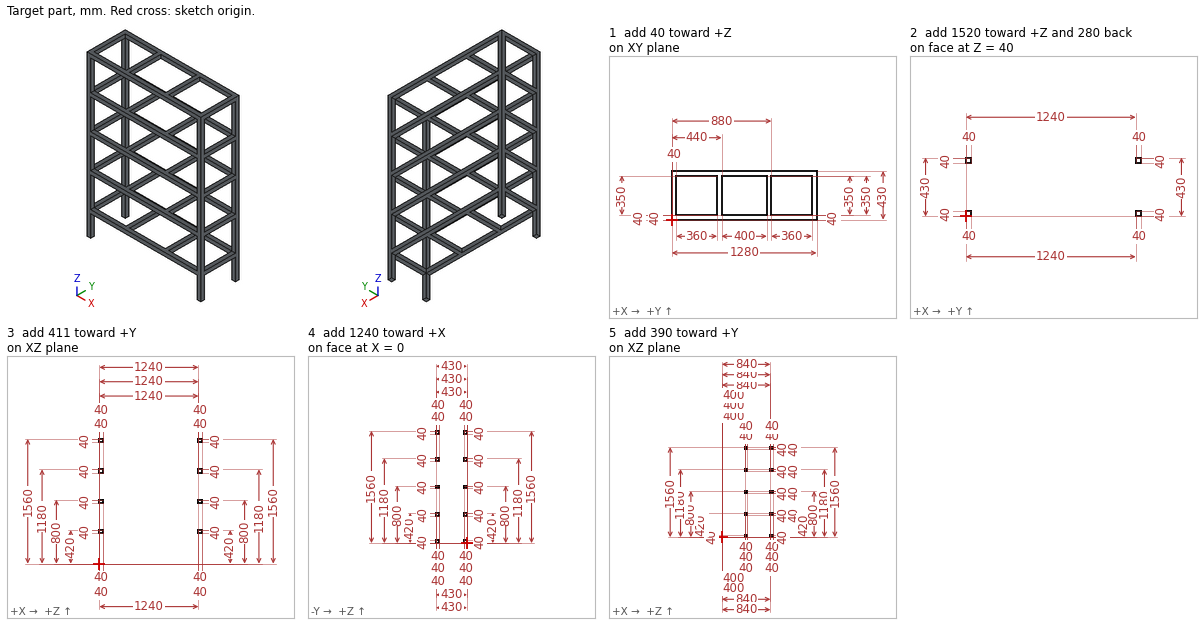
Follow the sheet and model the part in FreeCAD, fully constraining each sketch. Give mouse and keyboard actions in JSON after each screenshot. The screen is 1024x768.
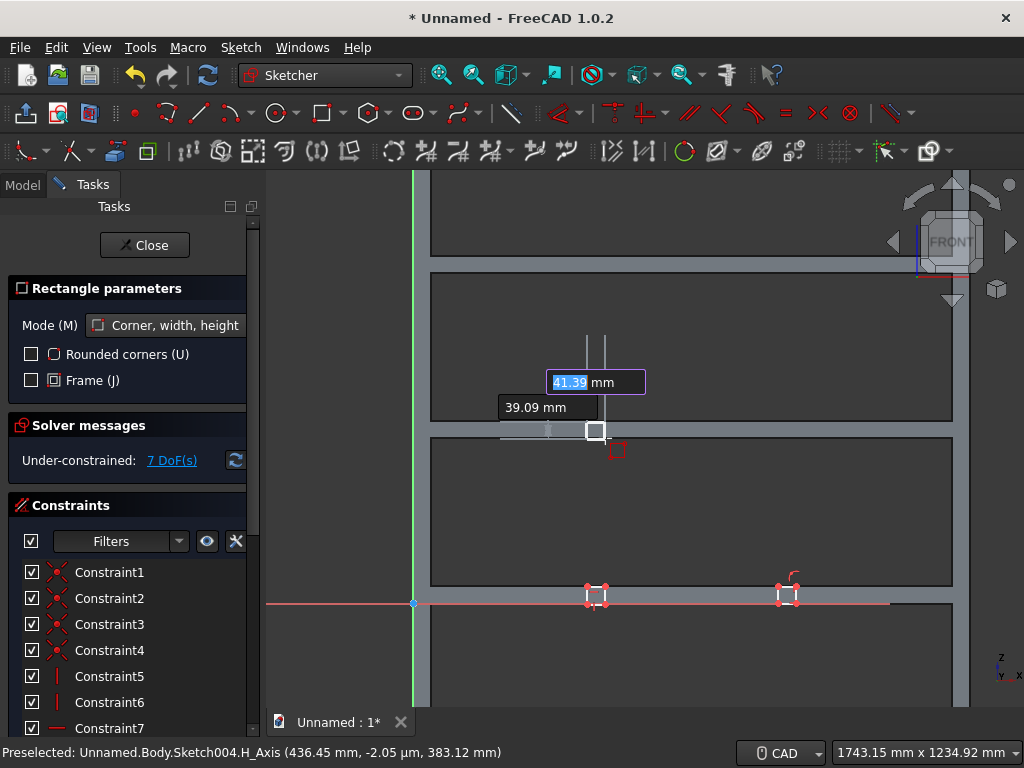
{"action": "type", "text": "40"}
{"action": "key", "text": "Tab"}
{"action": "type", "text": "40"}
{"action": "key", "text": "Return"}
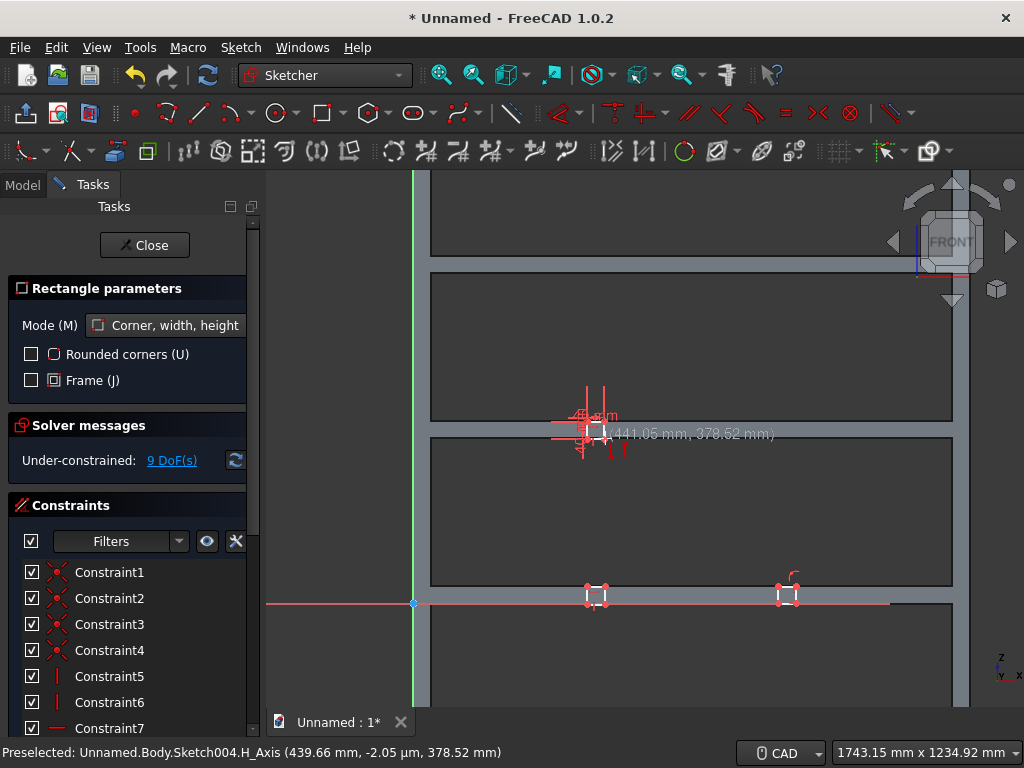
{"action": "left_click", "coordinate": [778, 421]}
{"action": "mouse_move", "coordinate": [796, 438]}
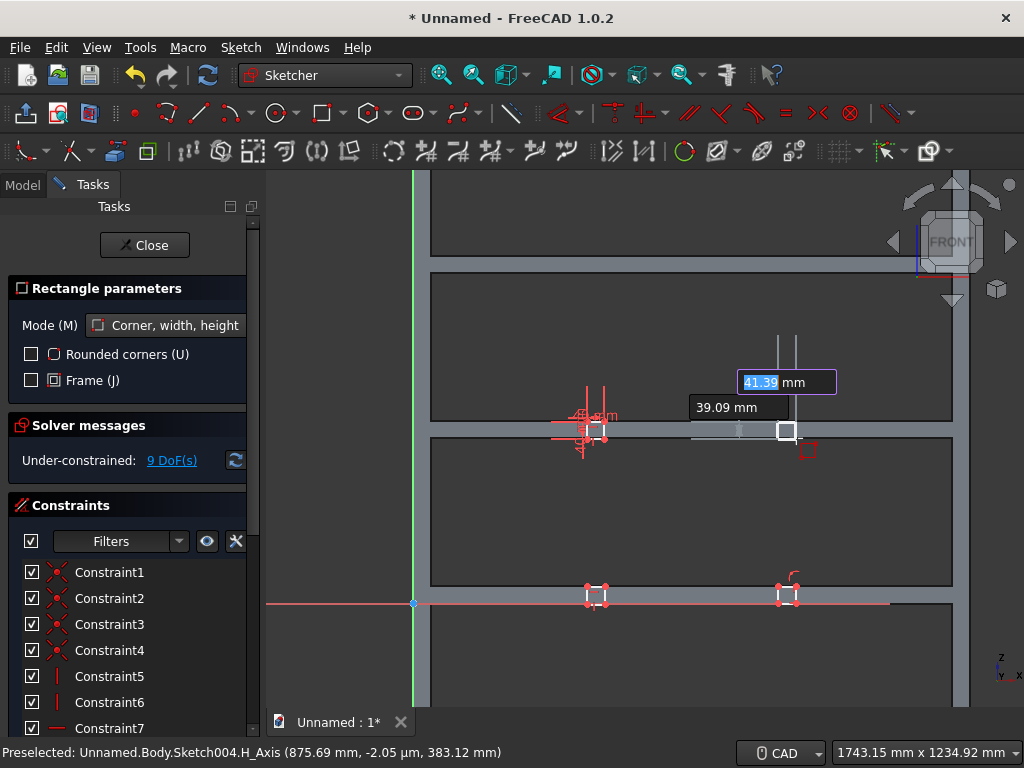
{"action": "type", "text": "40"}
{"action": "key", "text": "Tab"}
{"action": "type", "text": "40"}
{"action": "key", "text": "Return"}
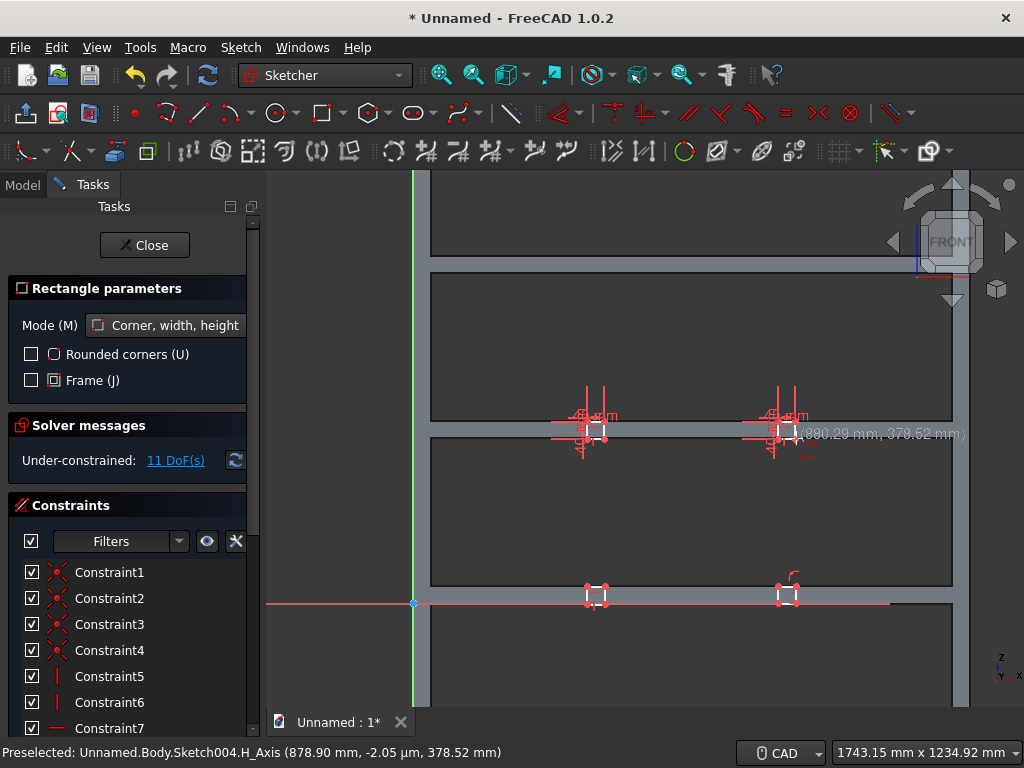
{"action": "left_click", "coordinate": [587, 256]}
{"action": "mouse_move", "coordinate": [605, 273]}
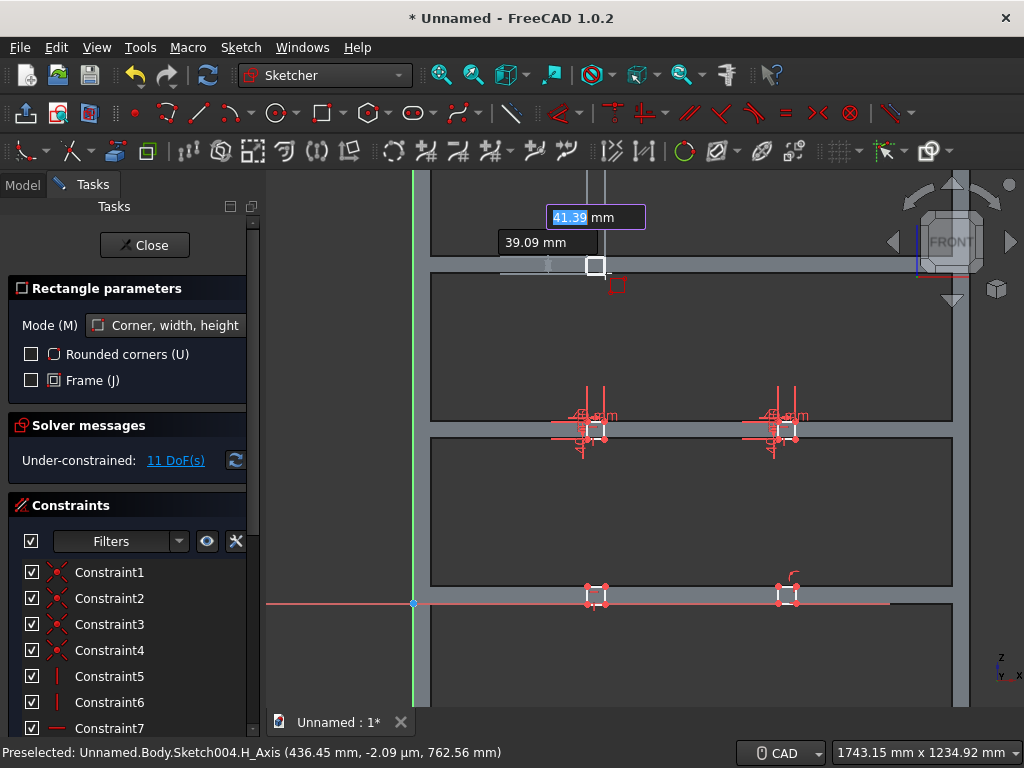
{"action": "type", "text": "40"}
{"action": "key", "text": "Tab"}
{"action": "type", "text": "40"}
{"action": "key", "text": "Return"}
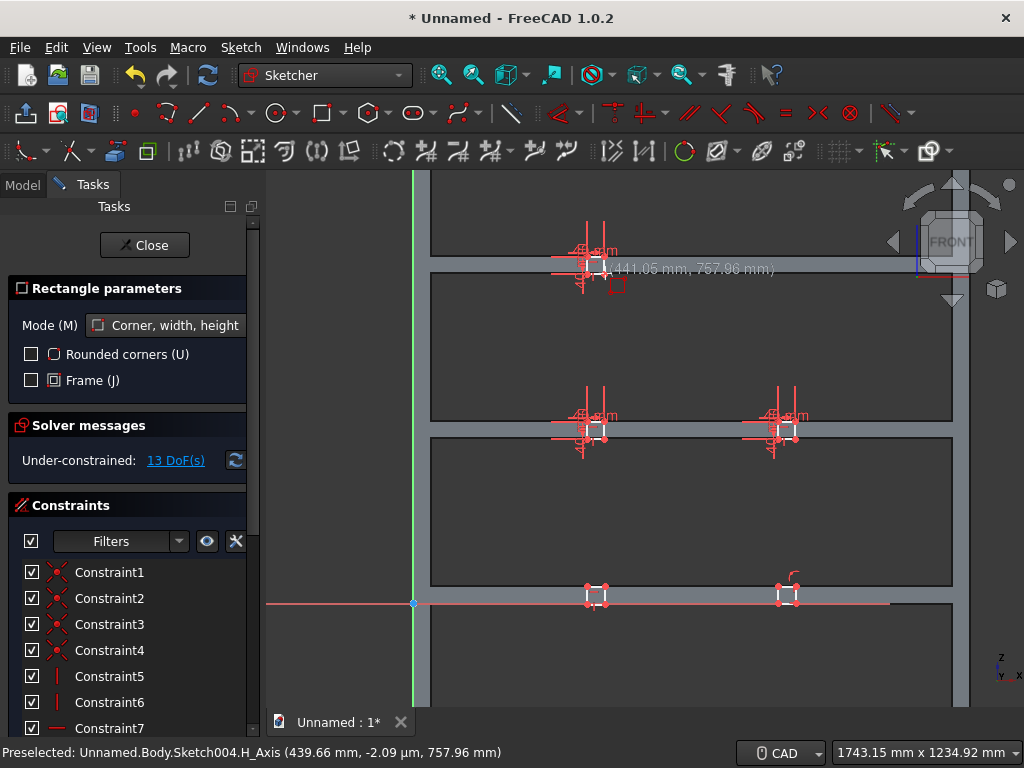
{"action": "left_click", "coordinate": [778, 256]}
{"action": "mouse_move", "coordinate": [796, 273]}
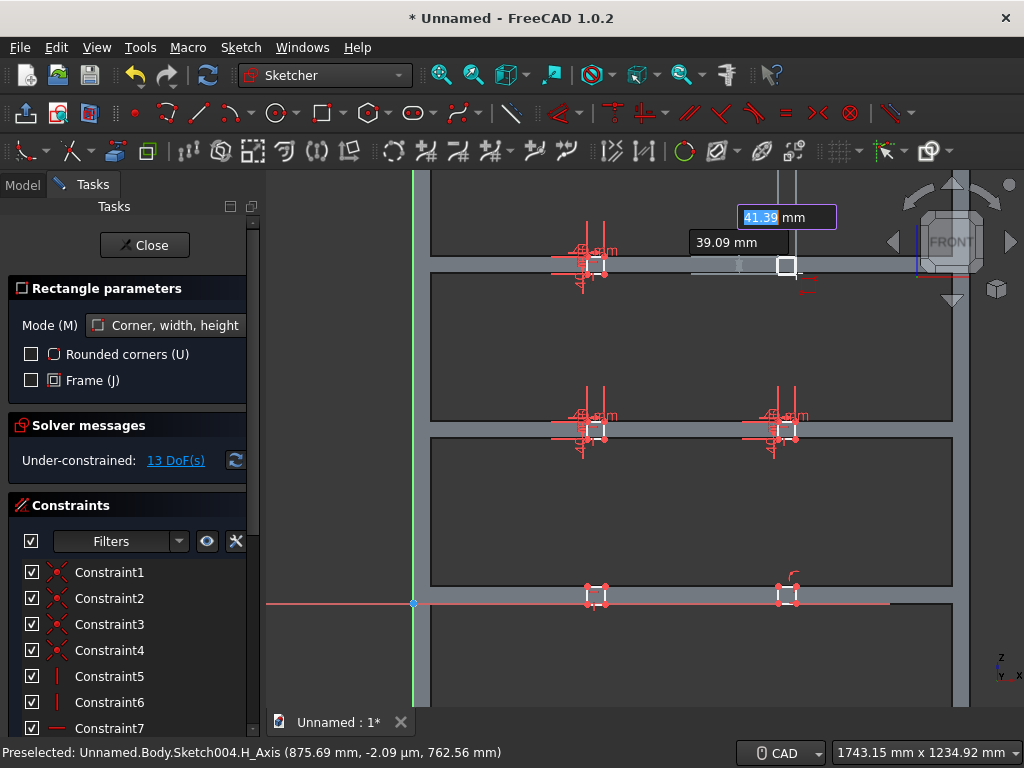
{"action": "type", "text": "40"}
{"action": "key", "text": "Tab"}
{"action": "type", "text": "40"}
{"action": "key", "text": "Return"}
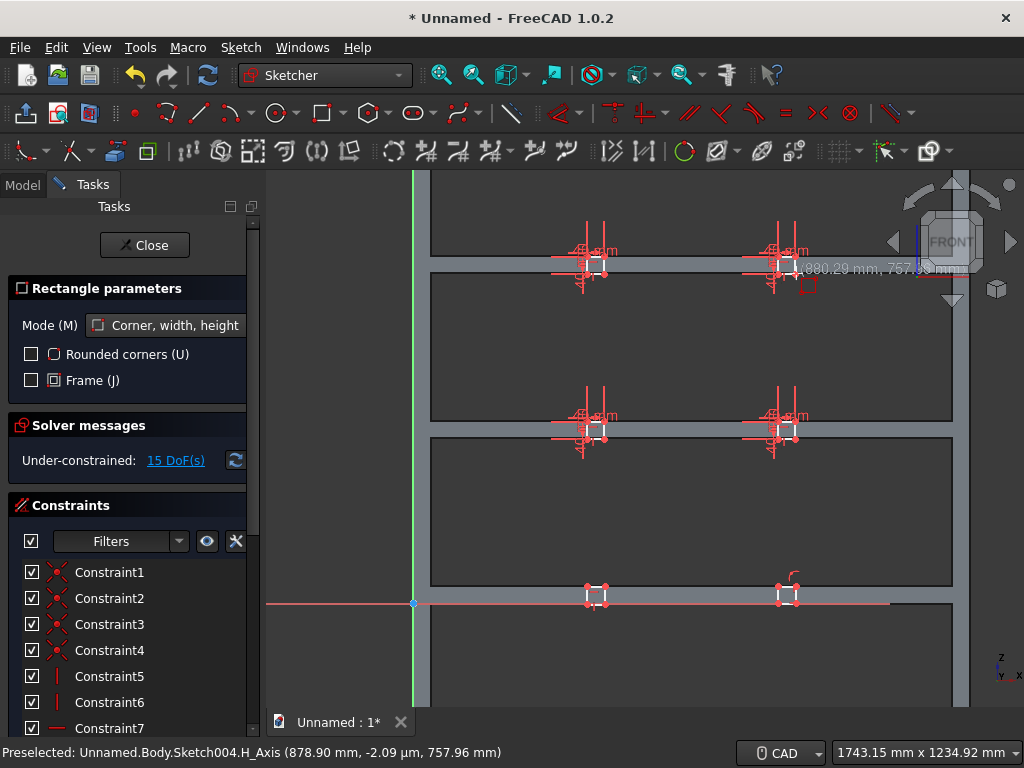
{"action": "scroll", "coordinate": [542, 650], "scroll_direction": "down", "scroll_amount": 3}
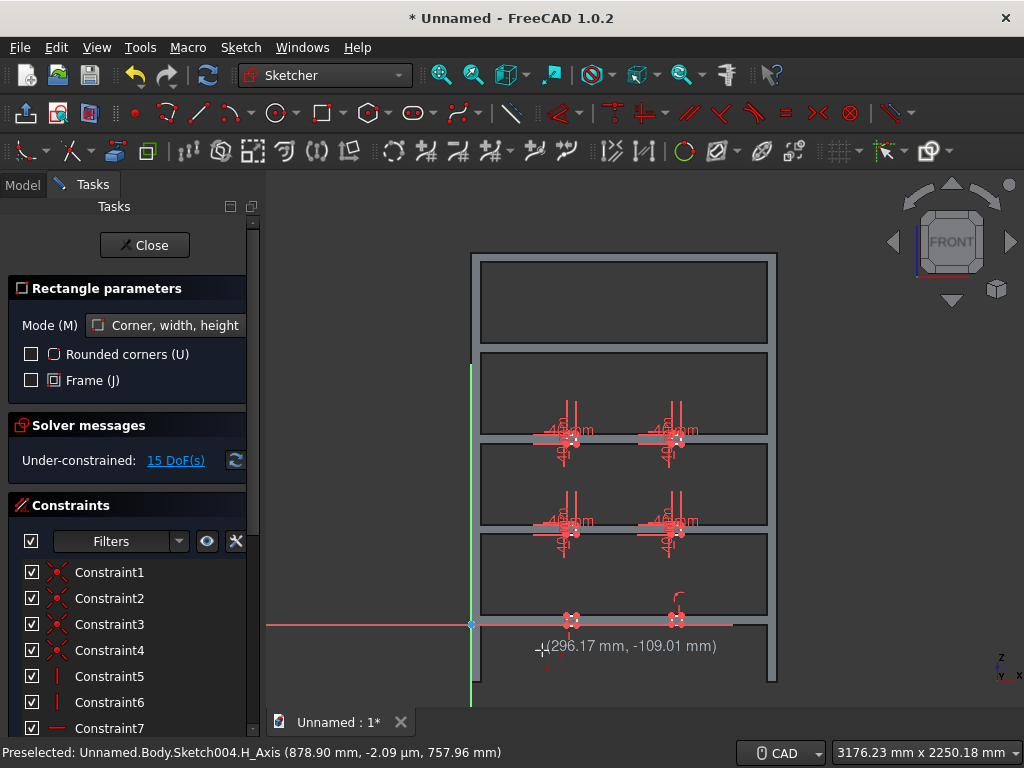
{"action": "scroll", "coordinate": [567, 343], "scroll_direction": "up", "scroll_amount": 3}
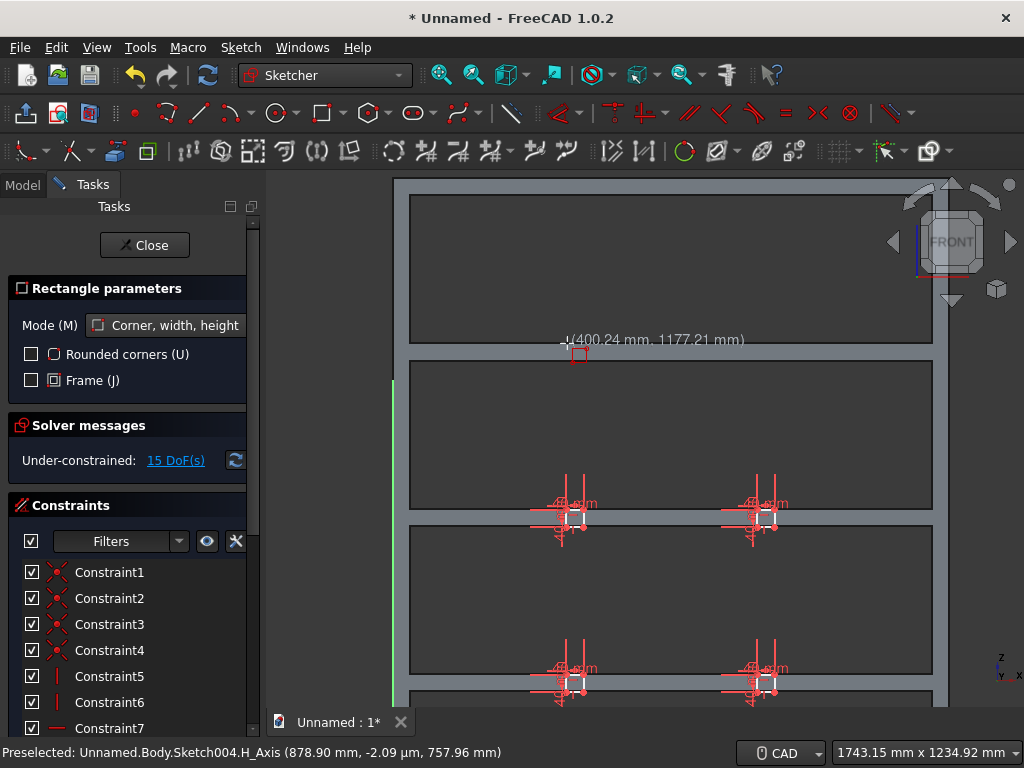
{"action": "left_click", "coordinate": [567, 343]}
{"action": "mouse_move", "coordinate": [584, 361]}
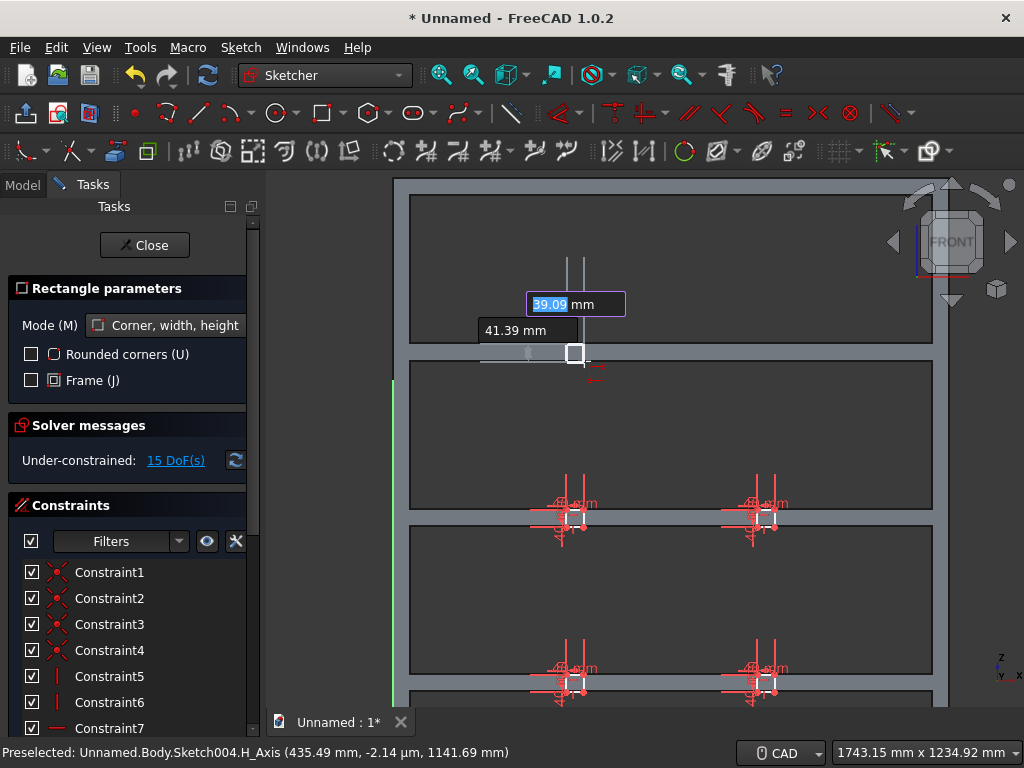
{"action": "type", "text": "40"}
{"action": "key", "text": "Tab"}
{"action": "type", "text": "40"}
{"action": "key", "text": "Return"}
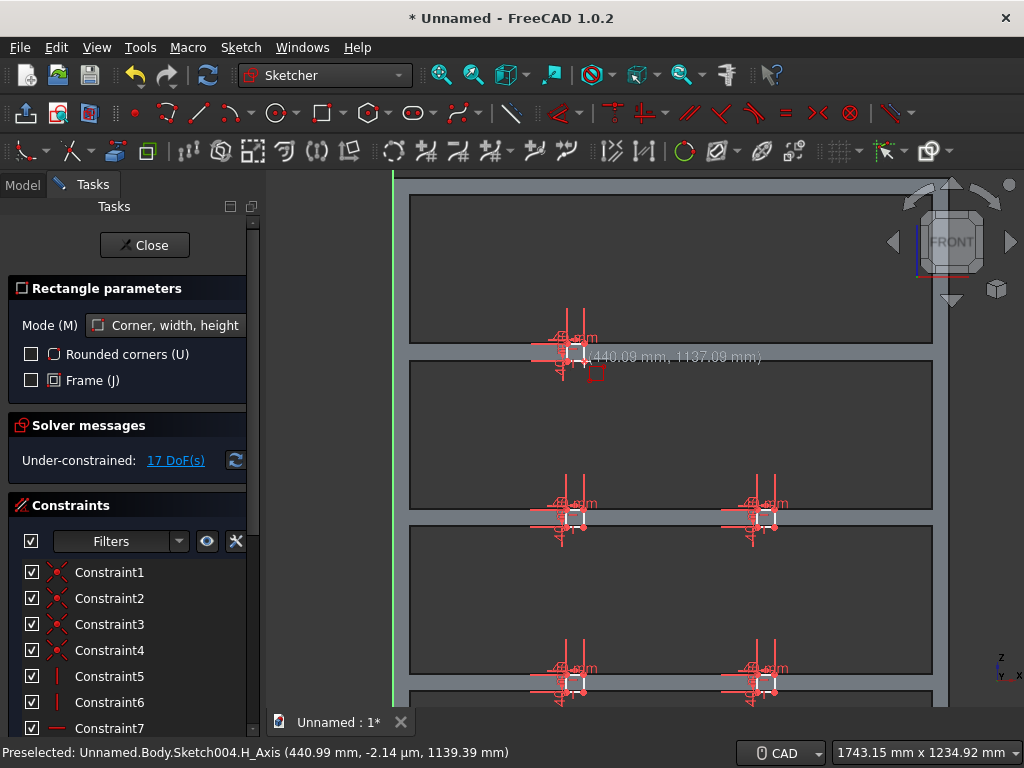
{"action": "left_click", "coordinate": [758, 343]}
{"action": "mouse_move", "coordinate": [775, 361]}